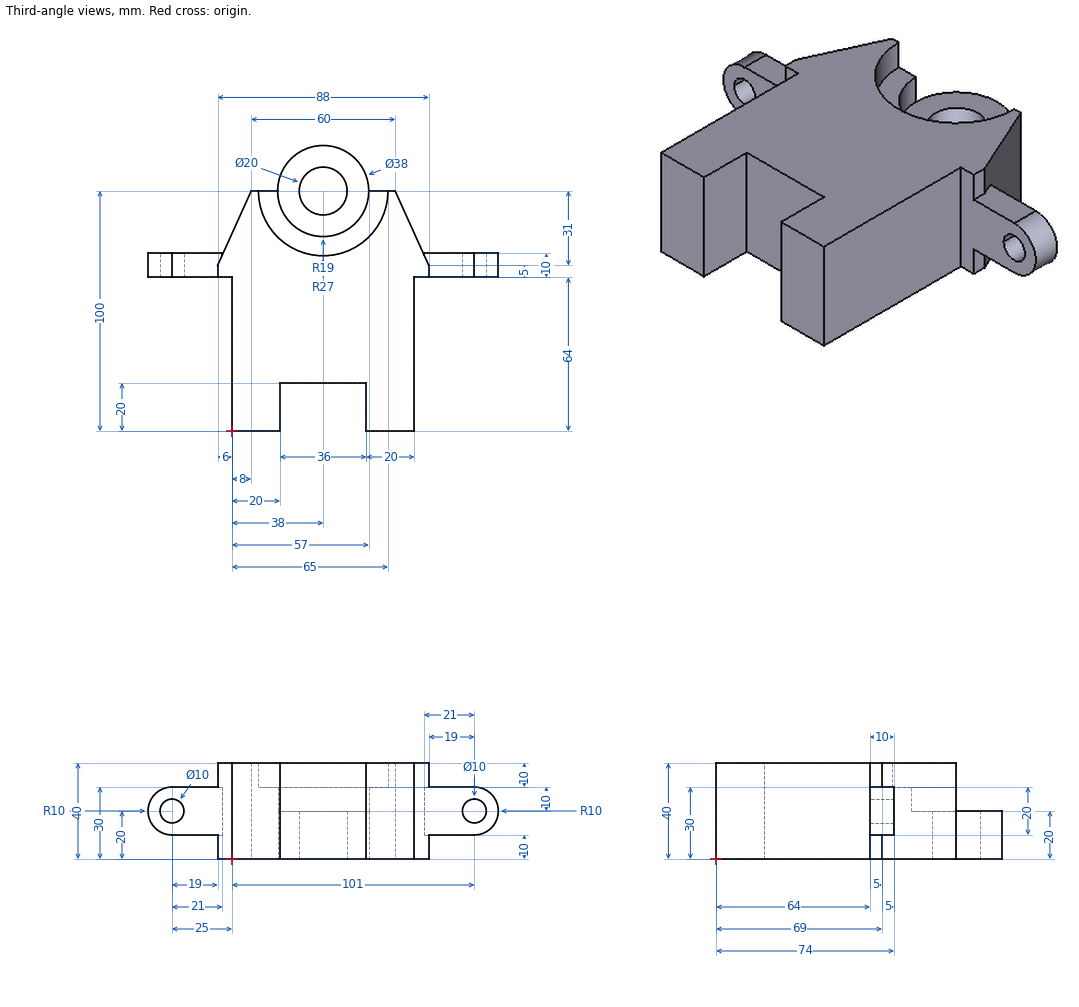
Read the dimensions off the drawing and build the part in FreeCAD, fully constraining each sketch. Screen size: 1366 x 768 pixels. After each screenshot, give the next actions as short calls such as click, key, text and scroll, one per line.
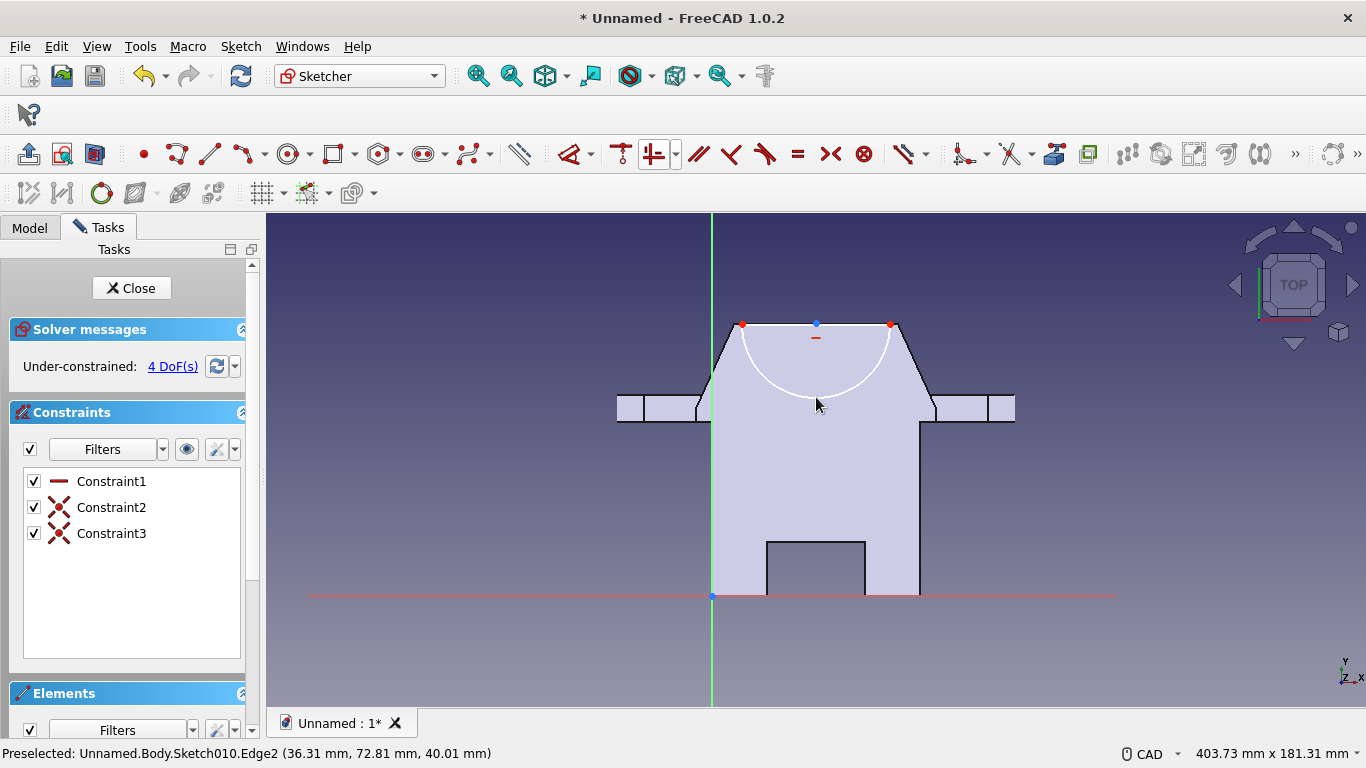
click(568, 154)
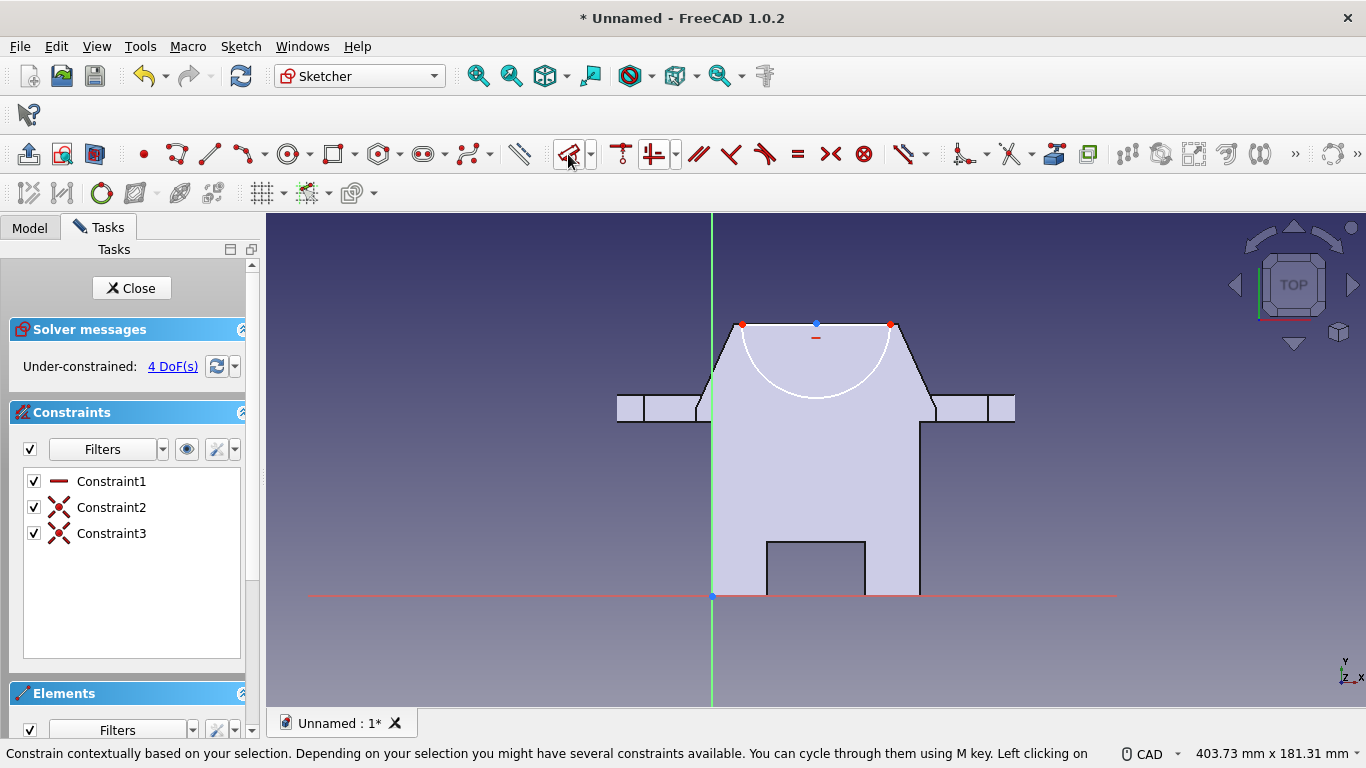
click(773, 384)
click(754, 410)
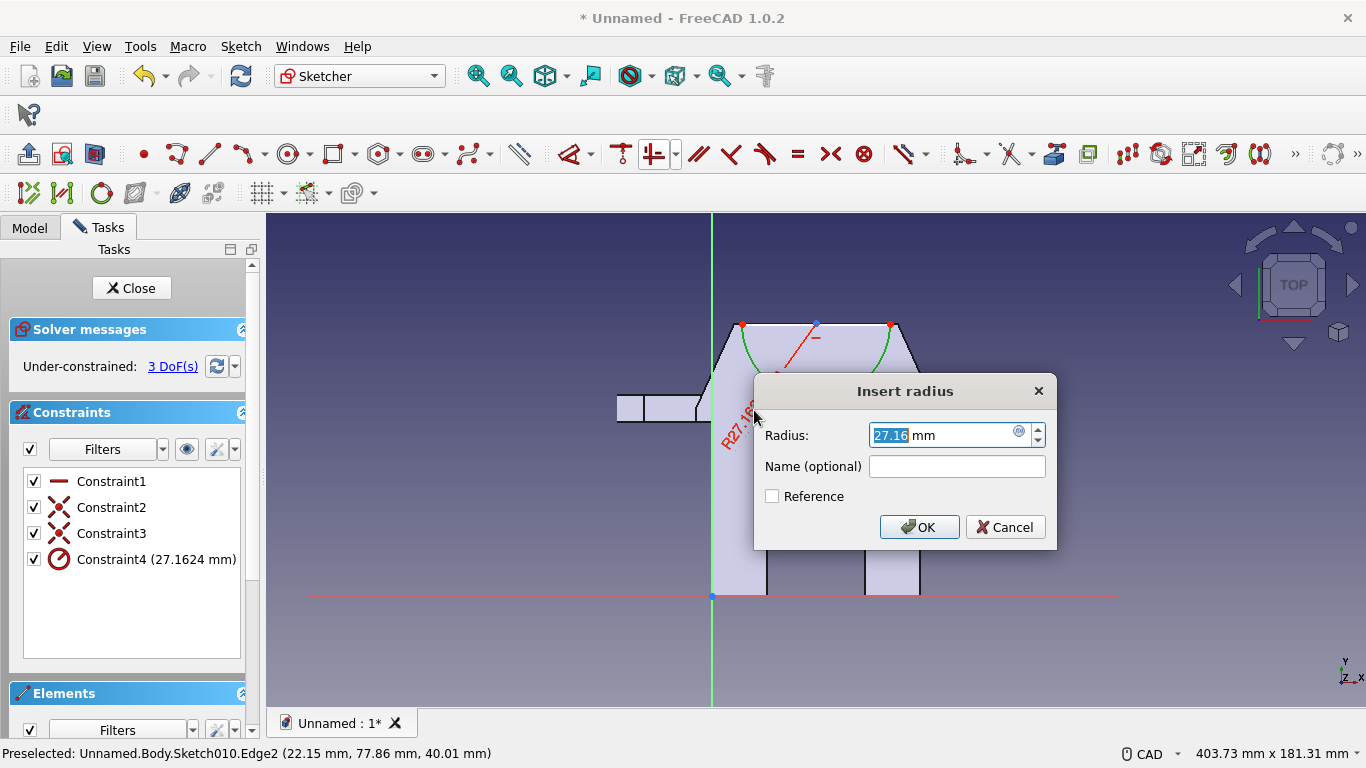
text(27)
key(Return)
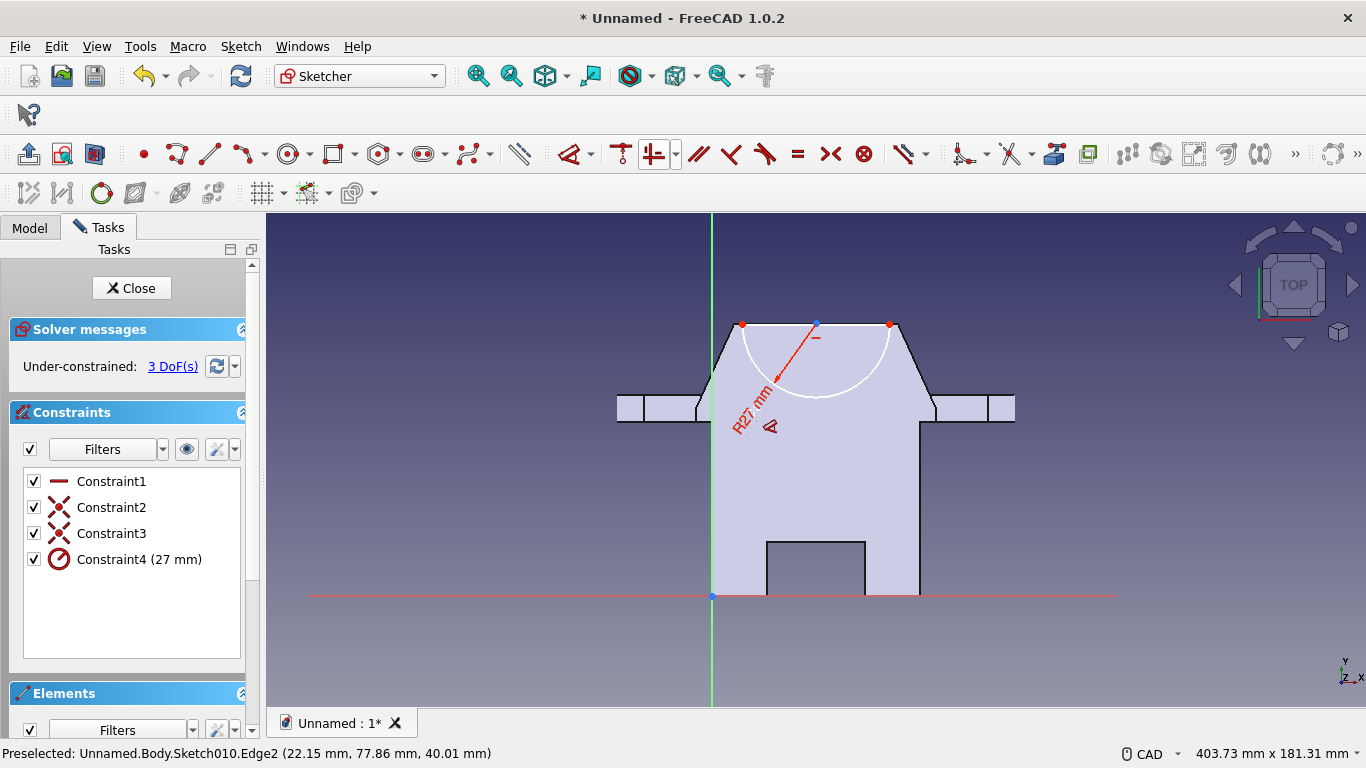
click(890, 325)
click(801, 630)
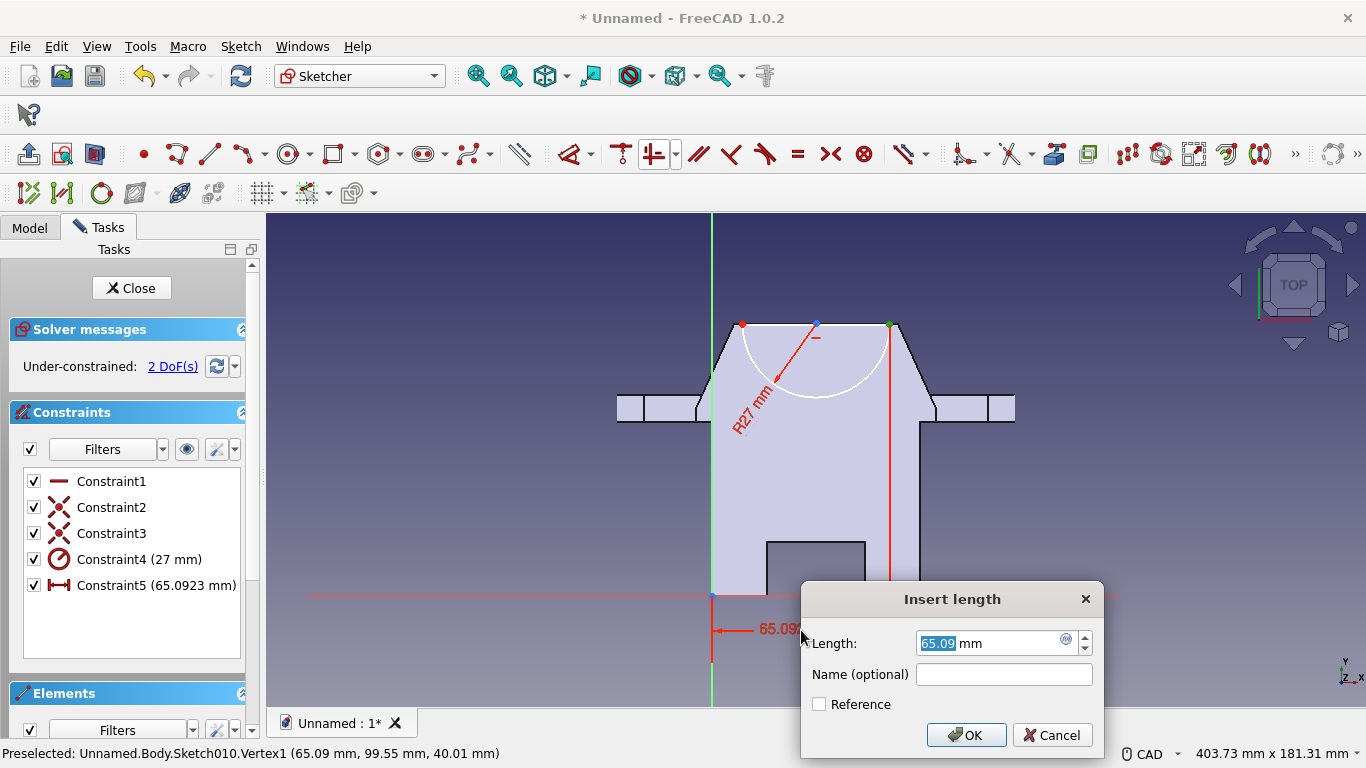
text(65)
key(Return)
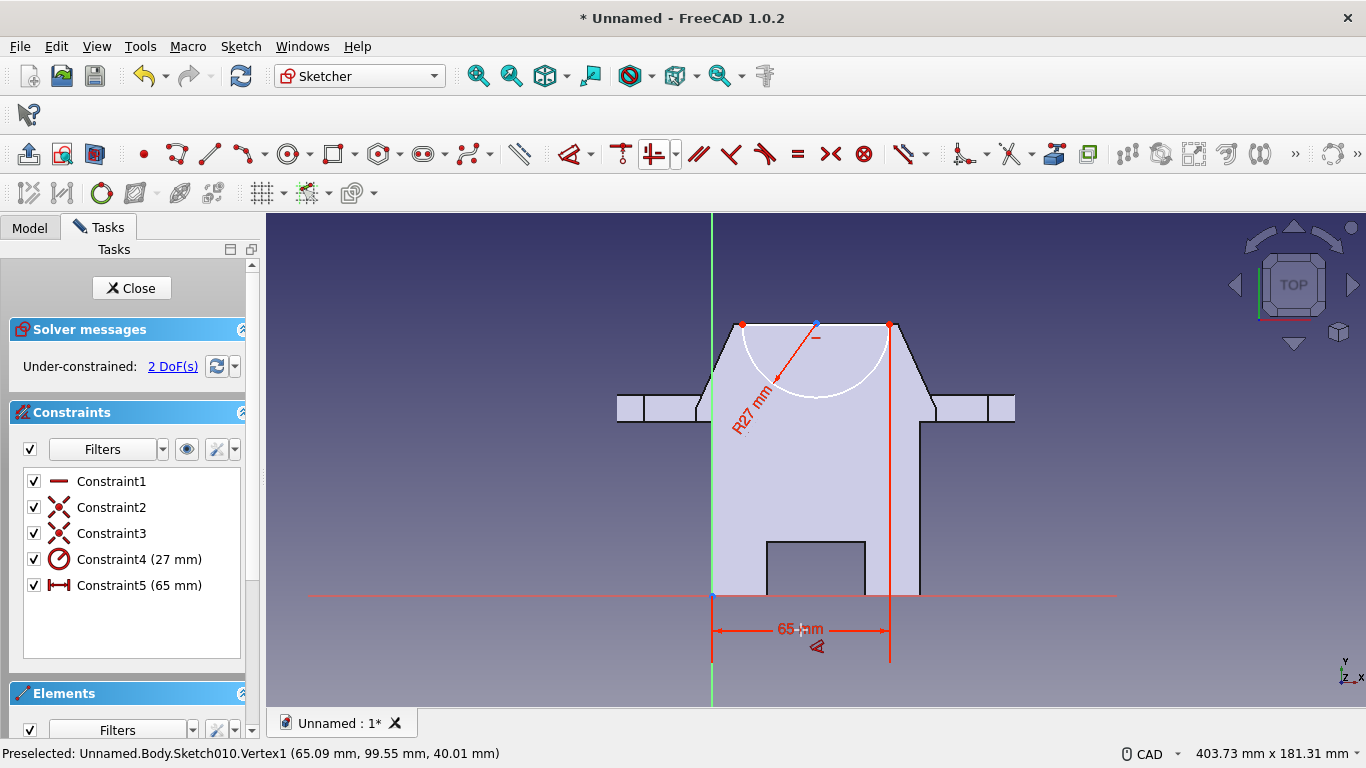
click(890, 325)
click(924, 461)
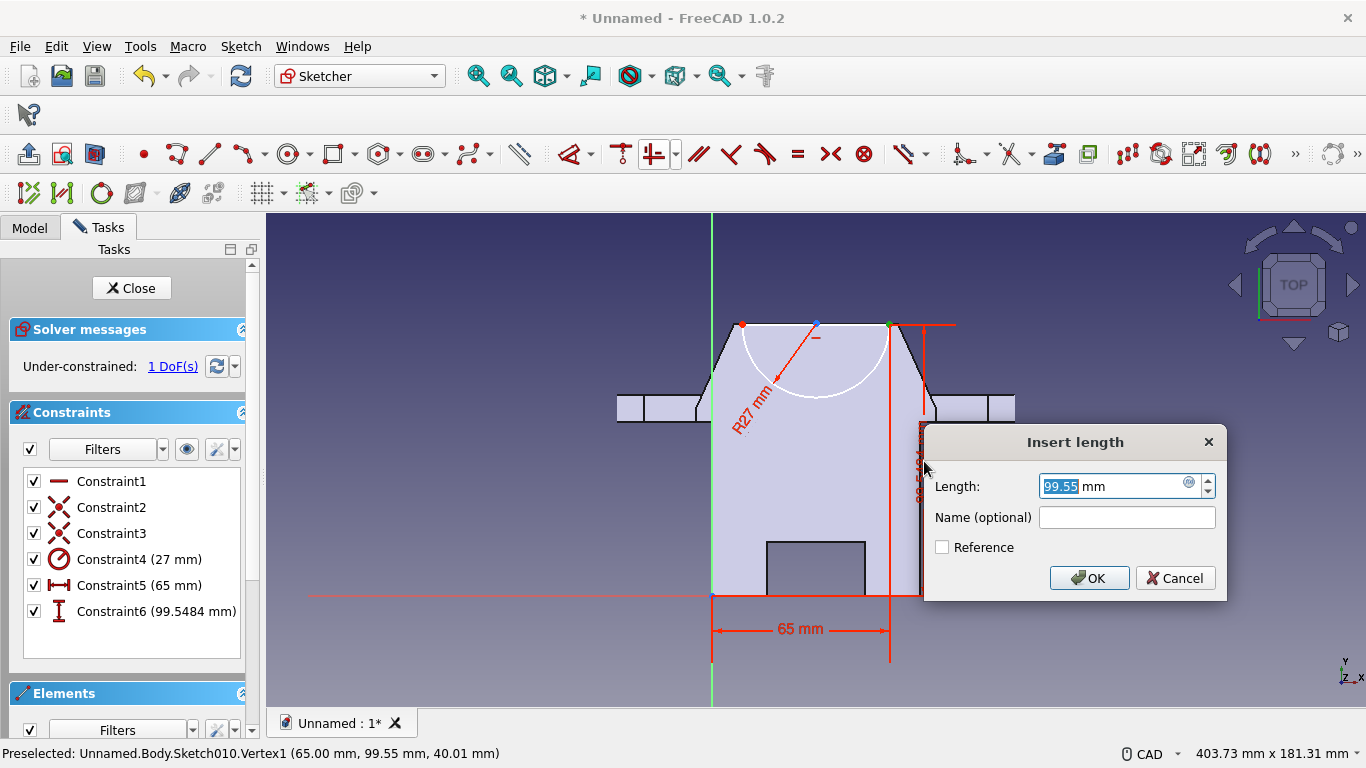
text(100)
key(Return)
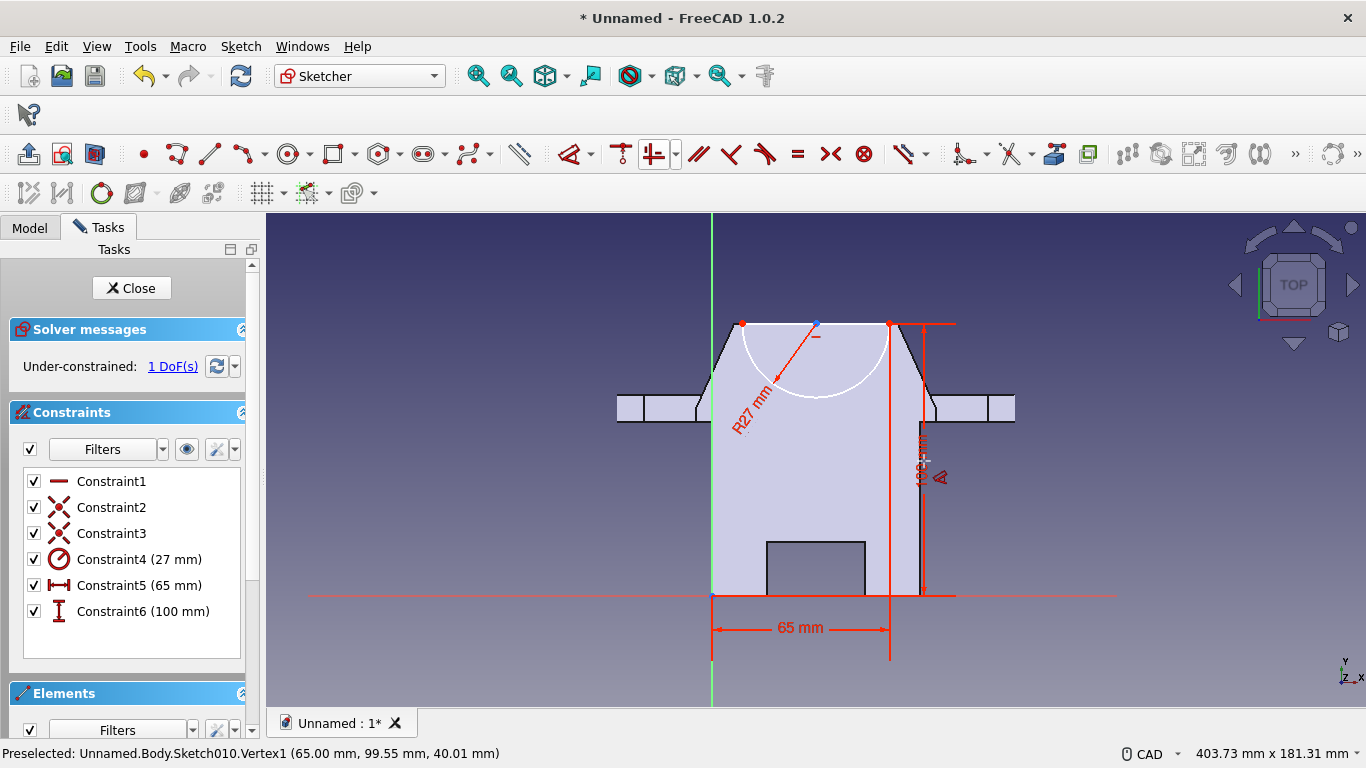
click(816, 324)
click(678, 460)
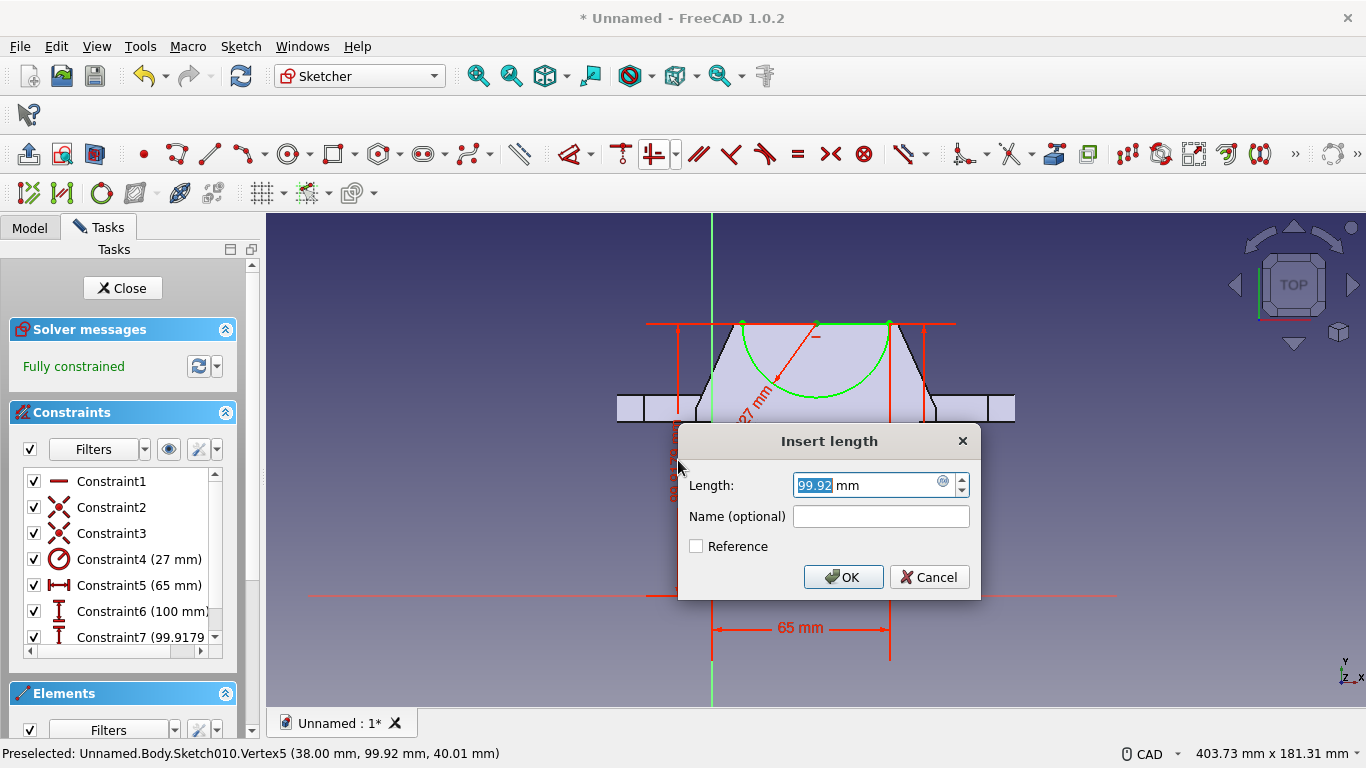
text(100)
key(Return)
key(Escape)